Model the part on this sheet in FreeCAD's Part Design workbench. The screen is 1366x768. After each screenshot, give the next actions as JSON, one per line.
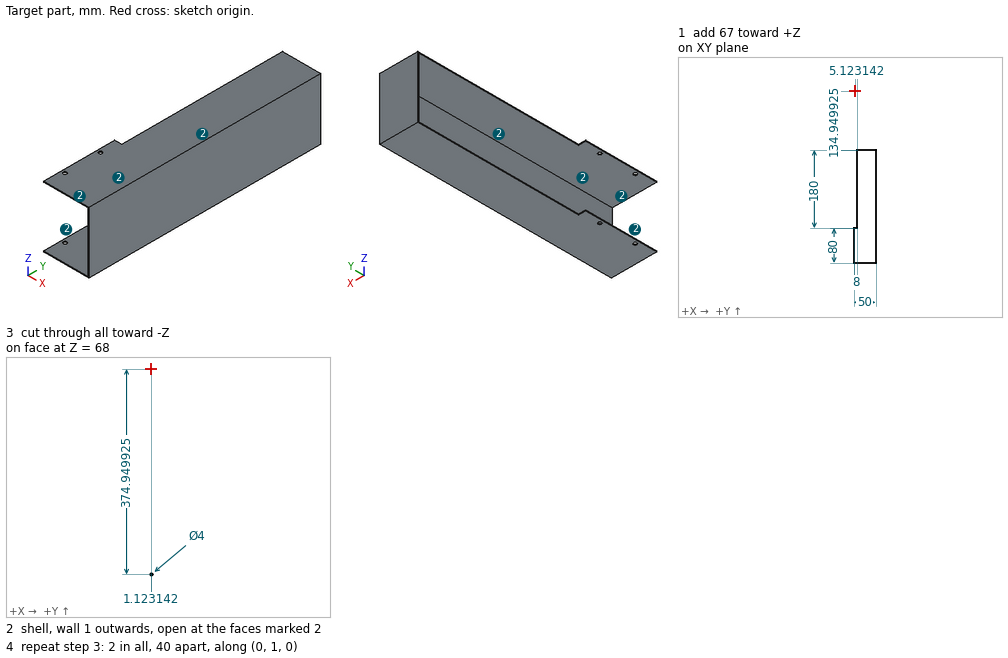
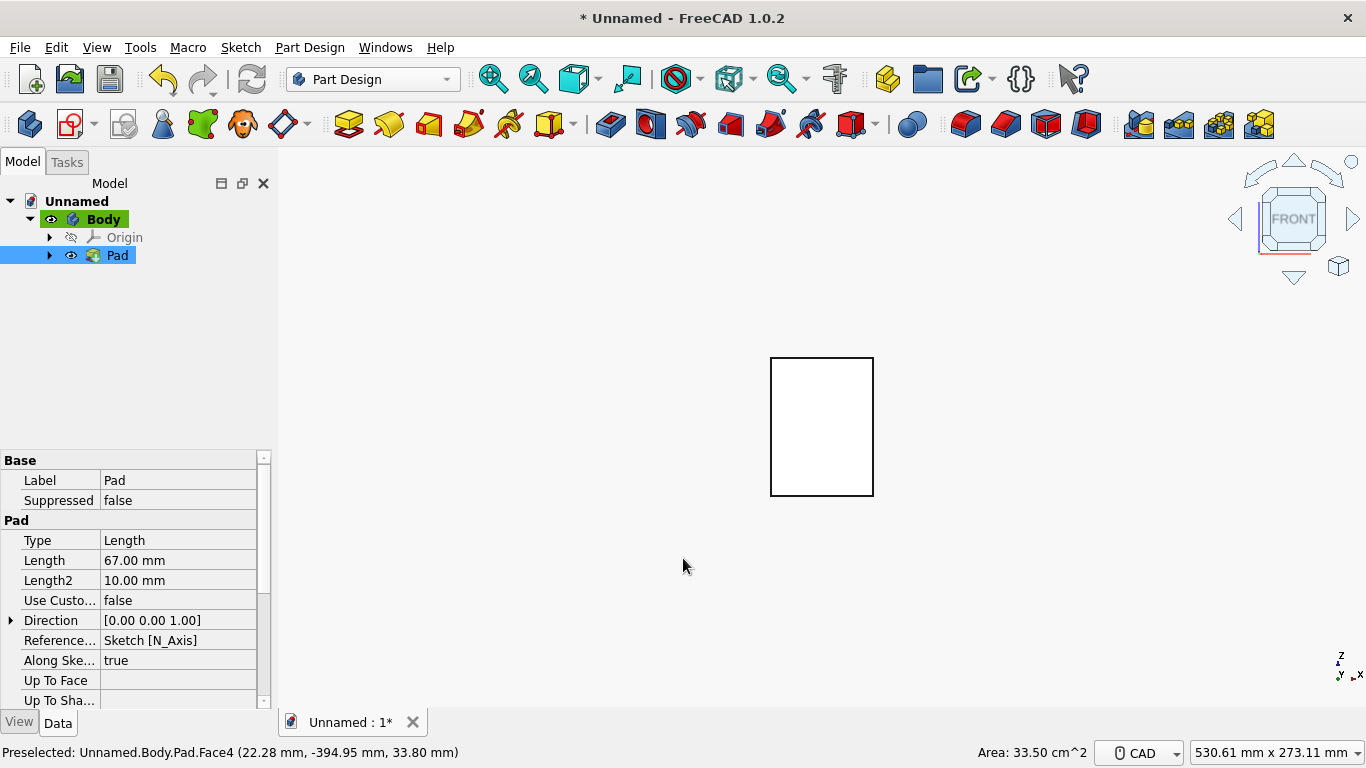
{"action": "left_click", "coordinate": [494, 80]}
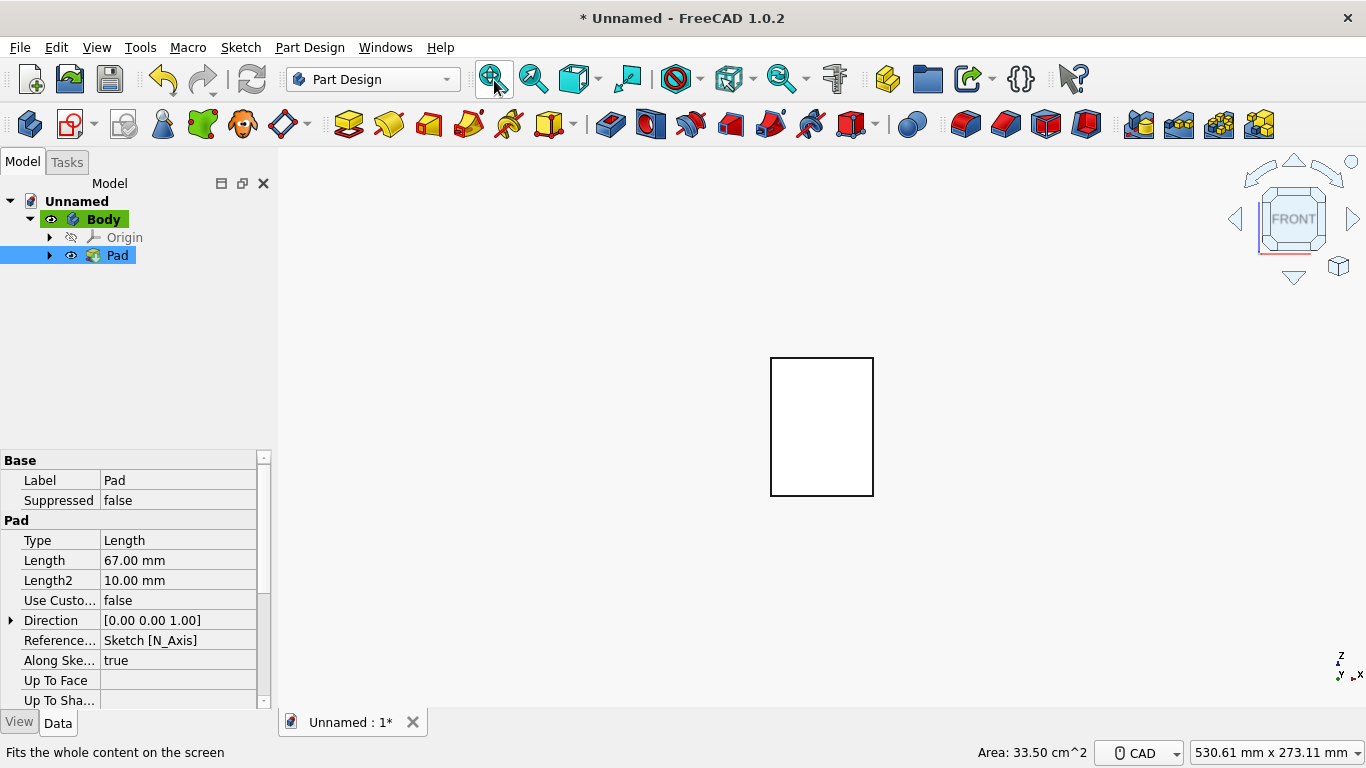
{"action": "key", "text": "3"}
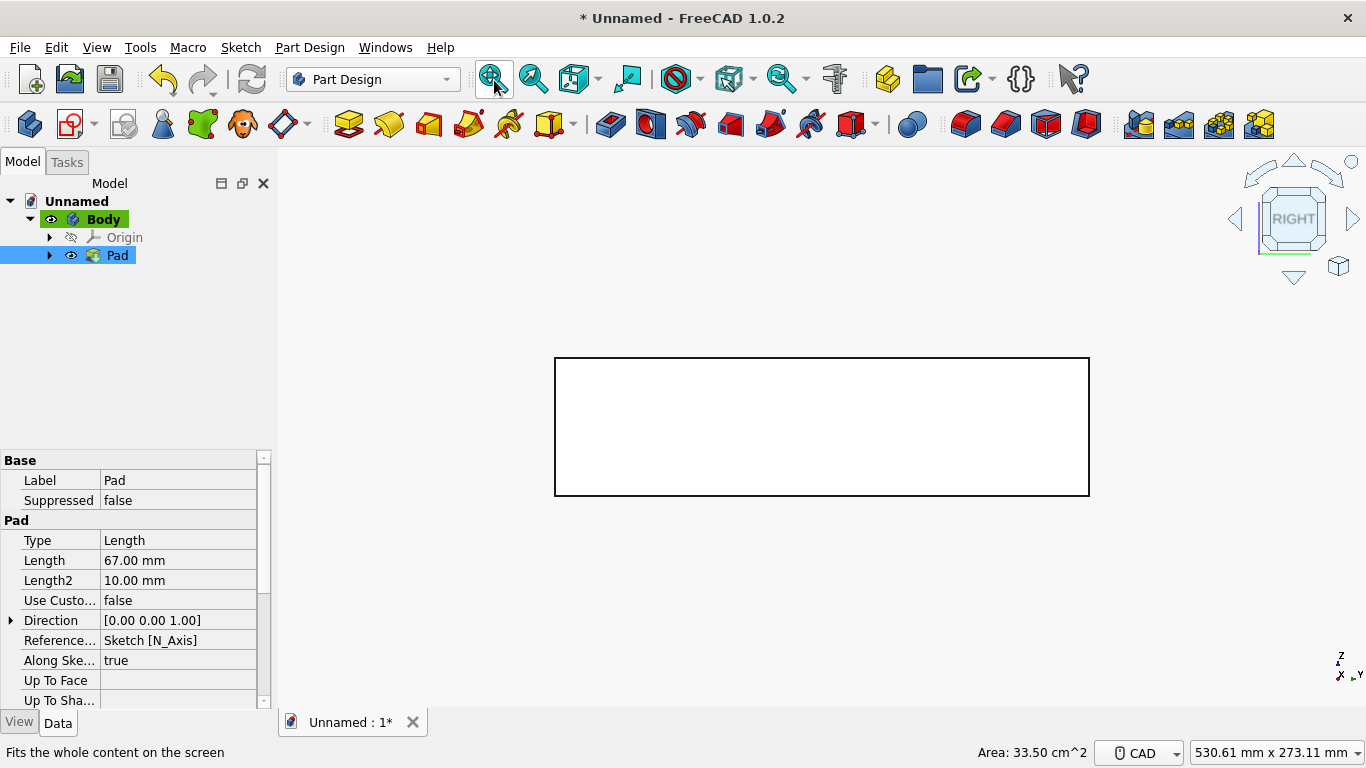
{"action": "key", "text": "5"}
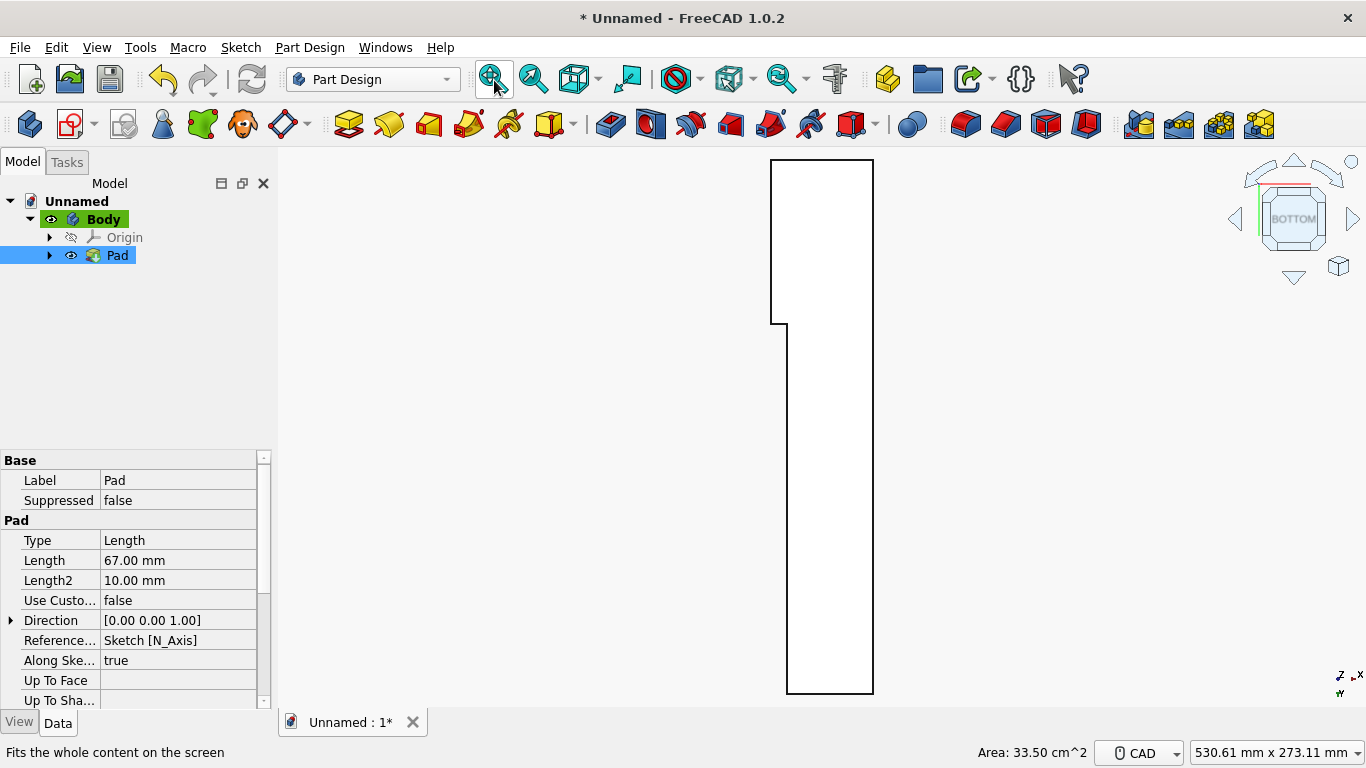
{"action": "key", "text": "4"}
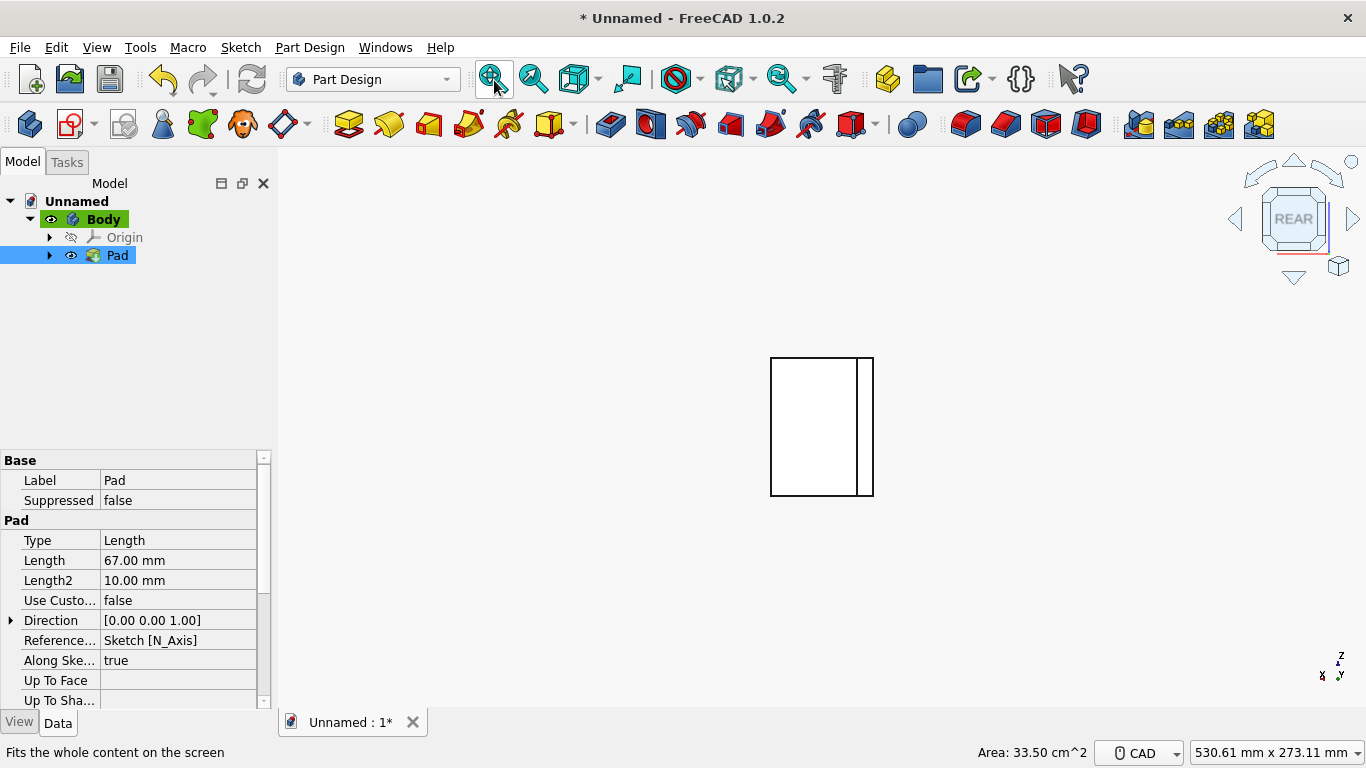
{"action": "left_click", "coordinate": [494, 80]}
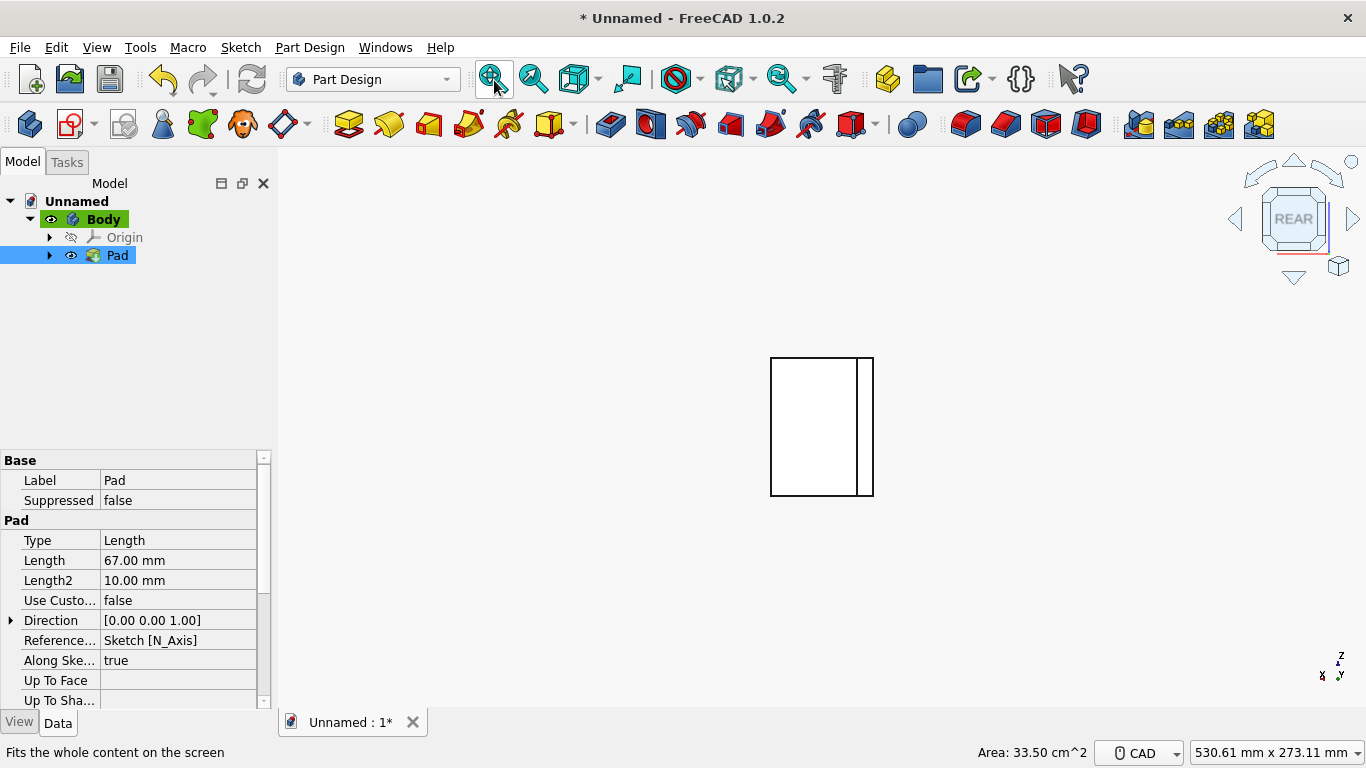
{"action": "left_click", "coordinate": [865, 367], "text": "ctrl"}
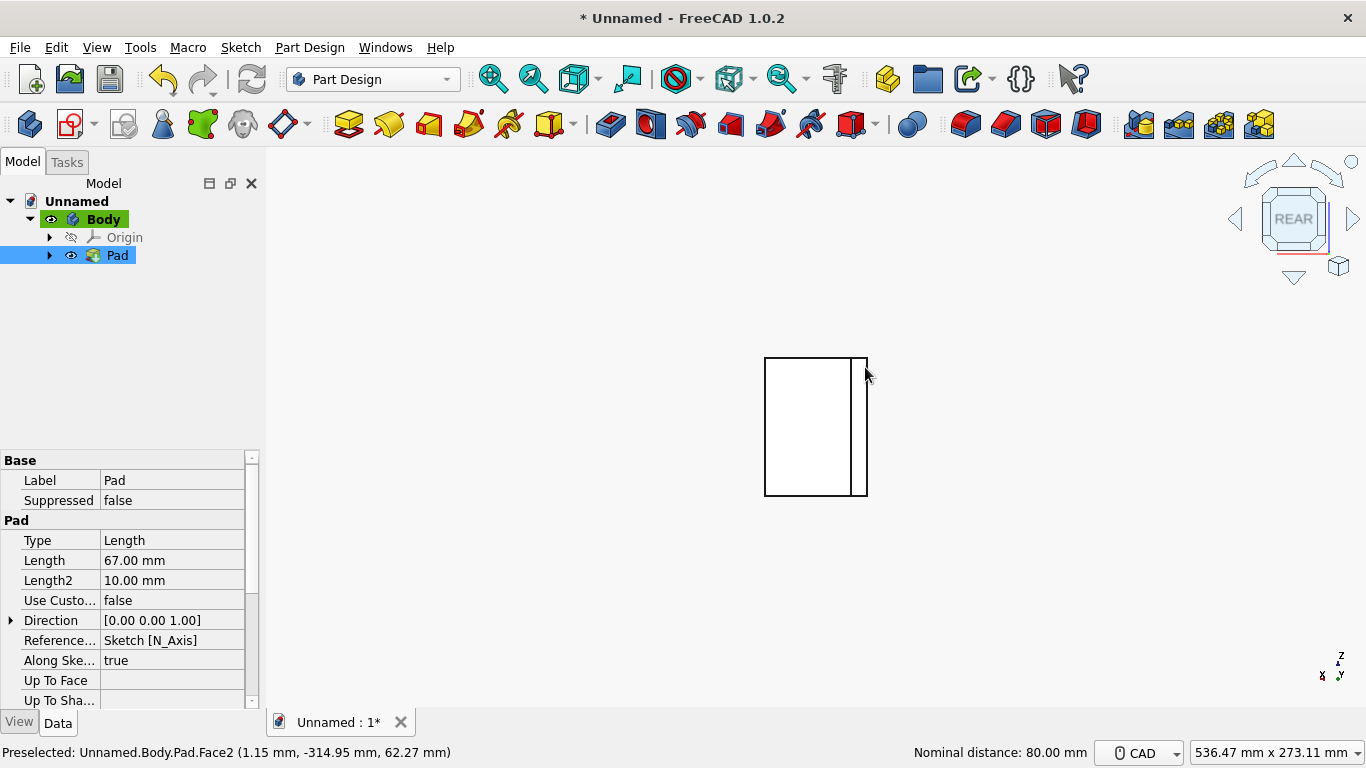
{"action": "key", "text": "6"}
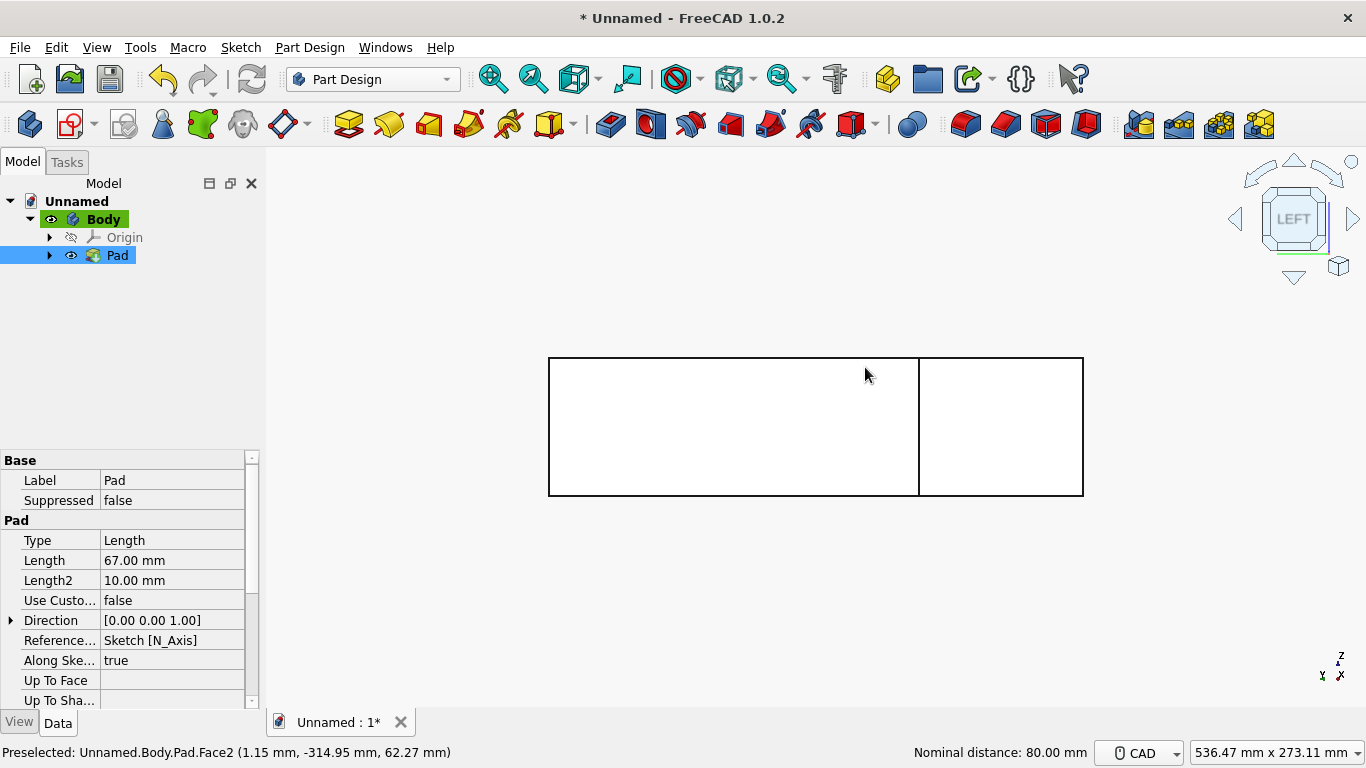
{"action": "left_click", "coordinate": [629, 426], "text": "ctrl"}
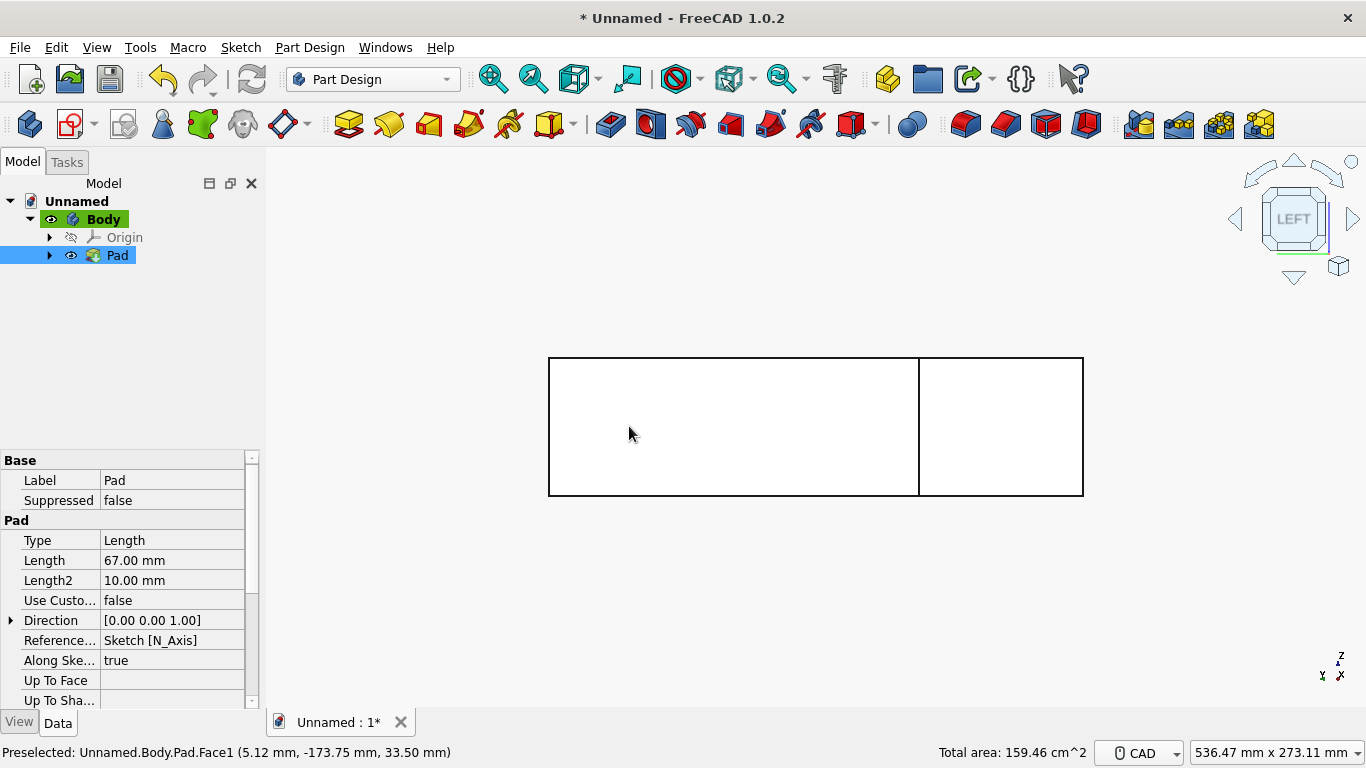
{"action": "left_click", "coordinate": [1001, 426], "text": "ctrl"}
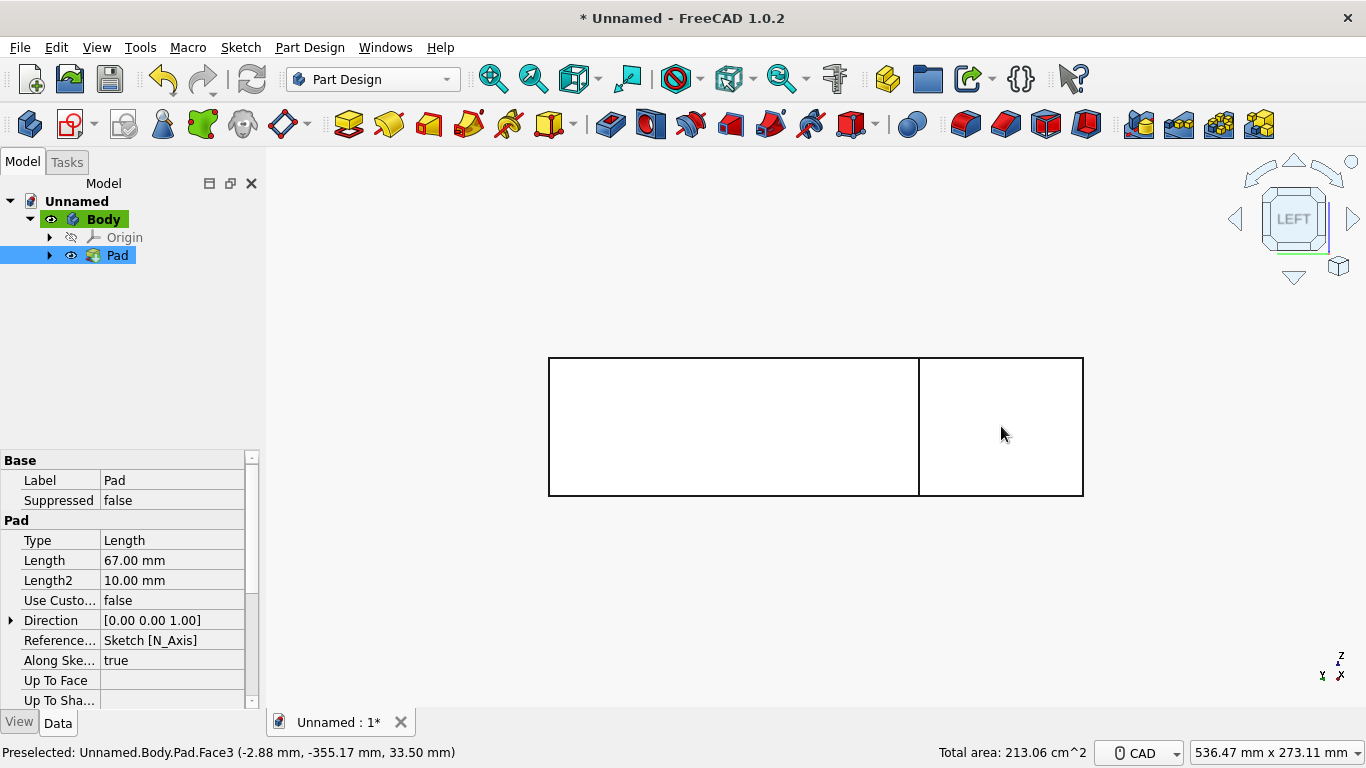
{"action": "left_click", "coordinate": [1086, 124]}